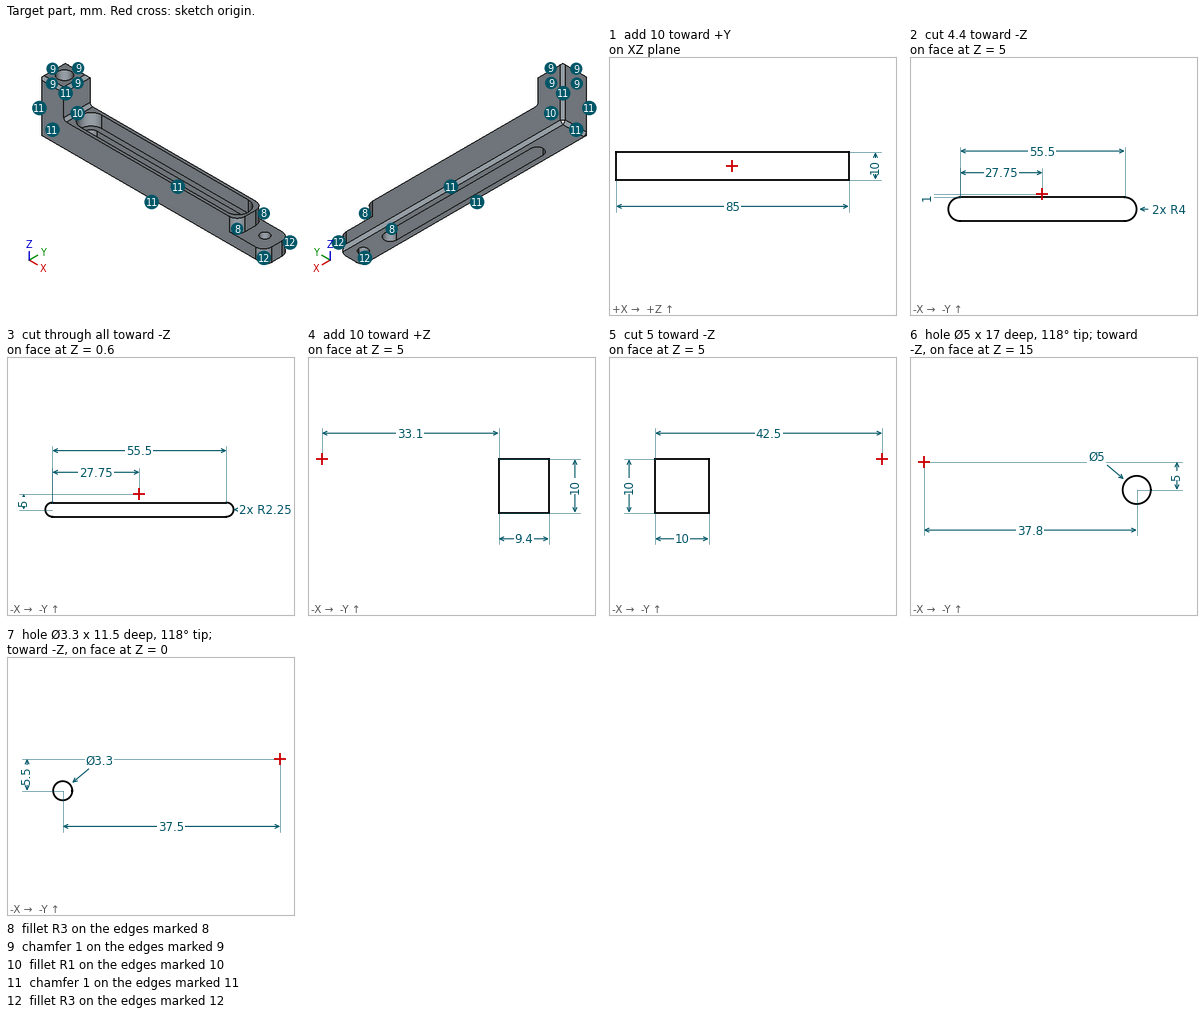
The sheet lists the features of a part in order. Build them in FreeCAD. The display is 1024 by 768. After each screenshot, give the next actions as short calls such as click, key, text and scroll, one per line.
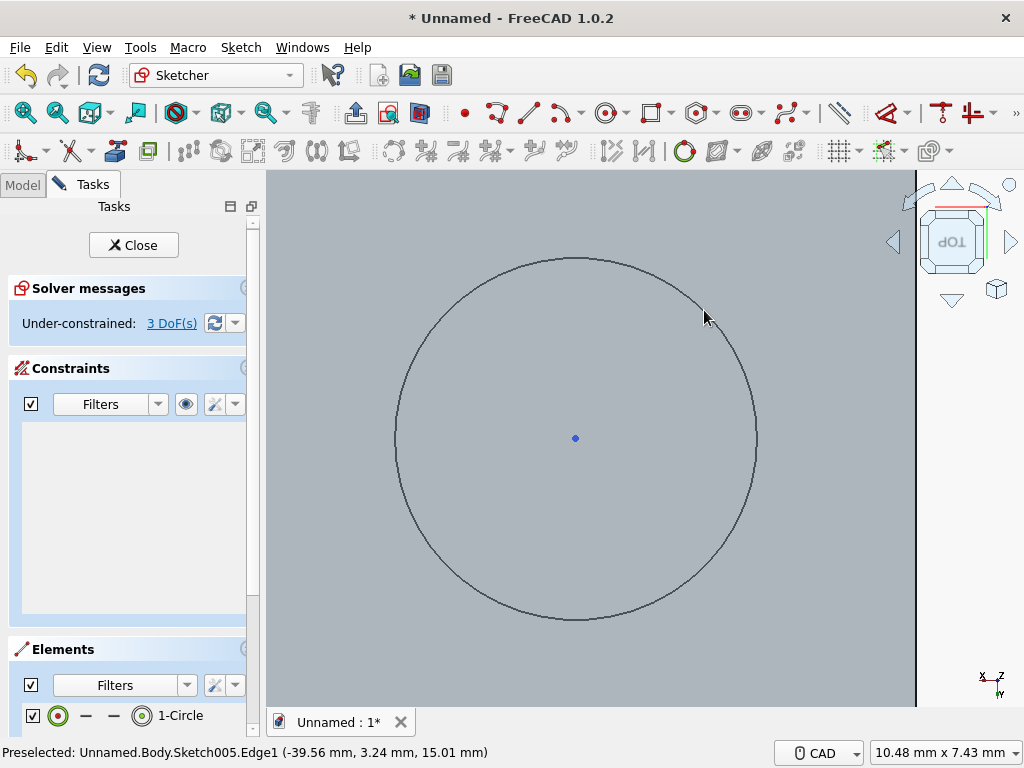
key(d)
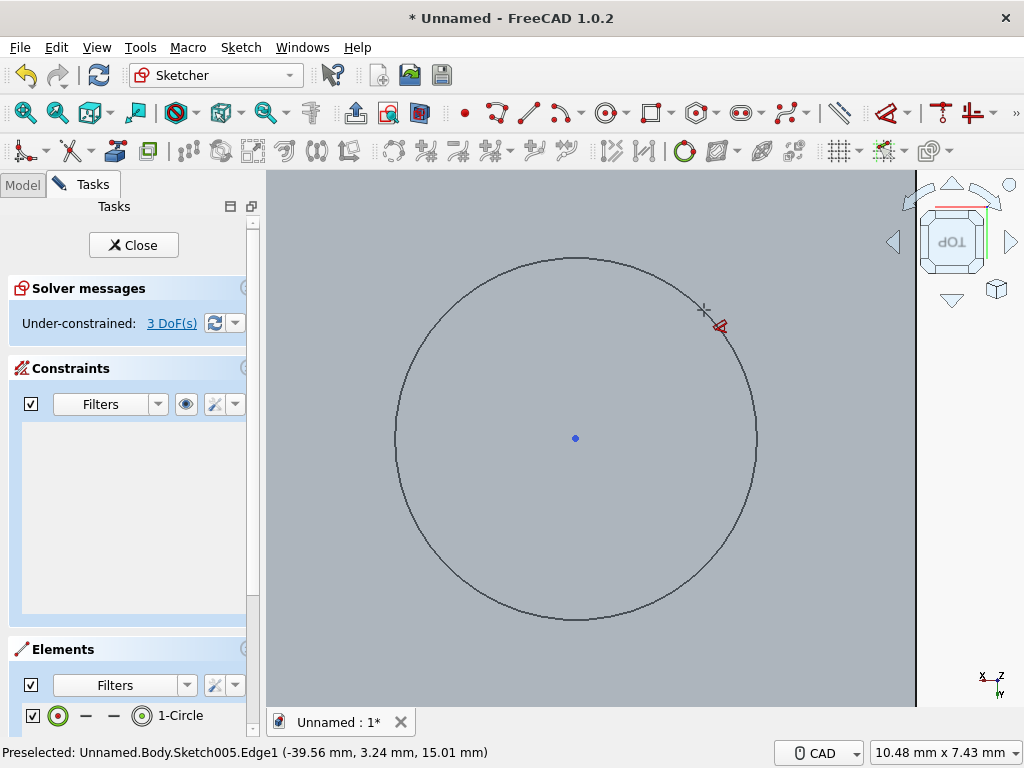
click(704, 311)
click(727, 288)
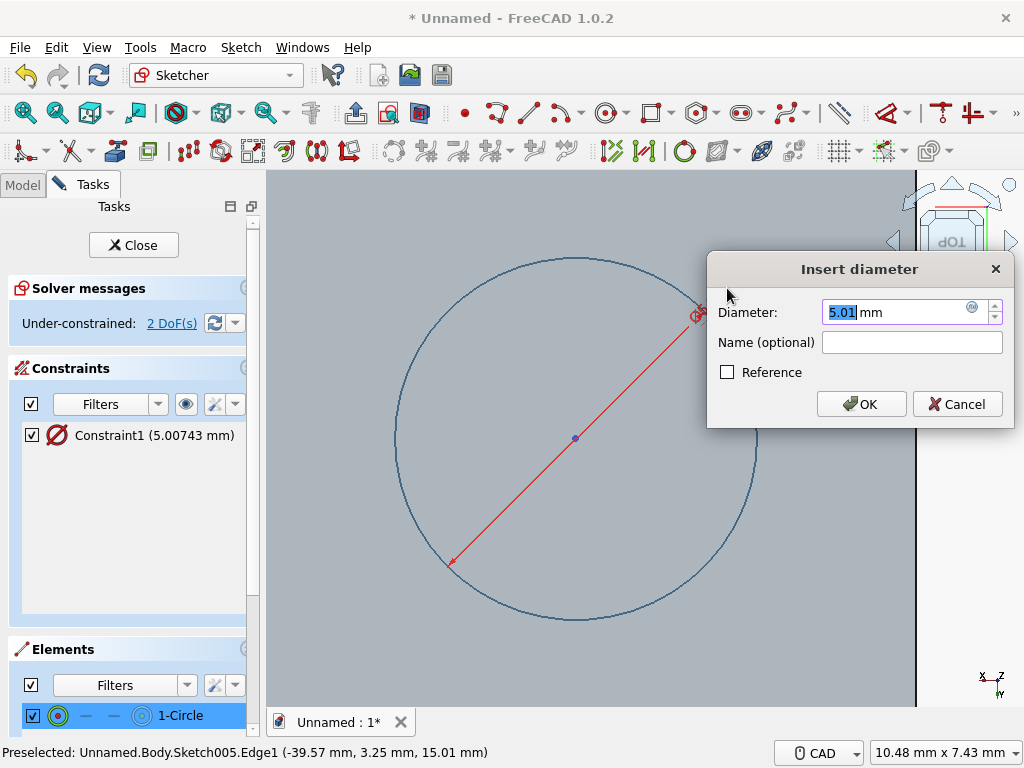
text(5)
key(Return)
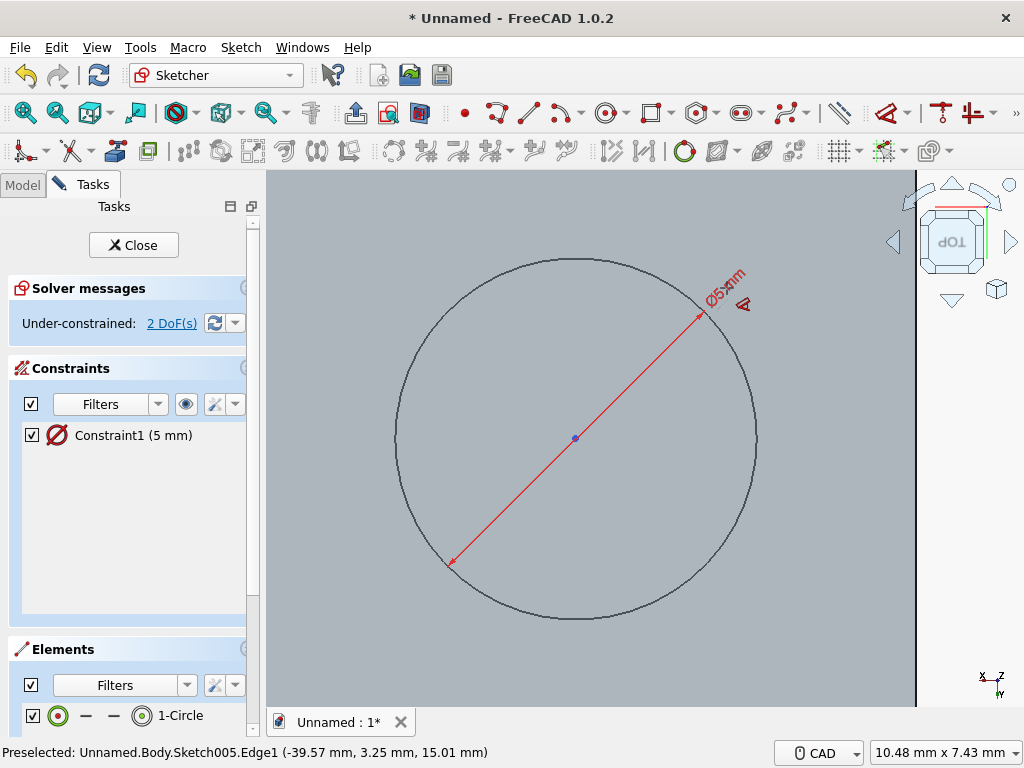
click(576, 439)
click(610, 318)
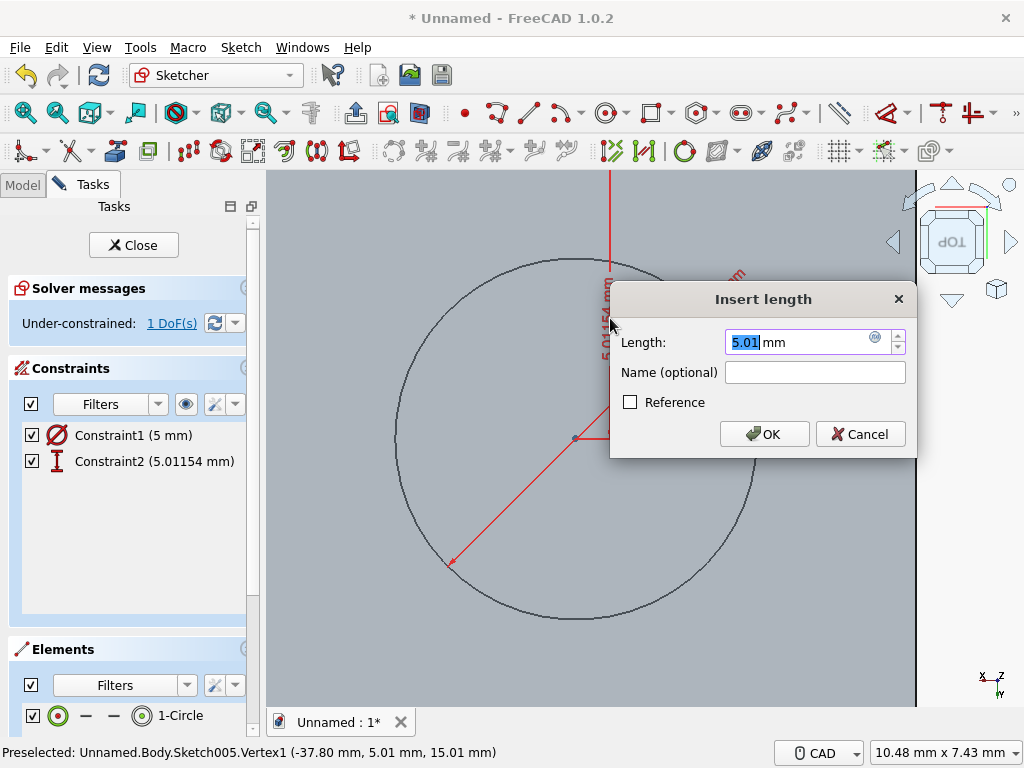
text(5)
key(Return)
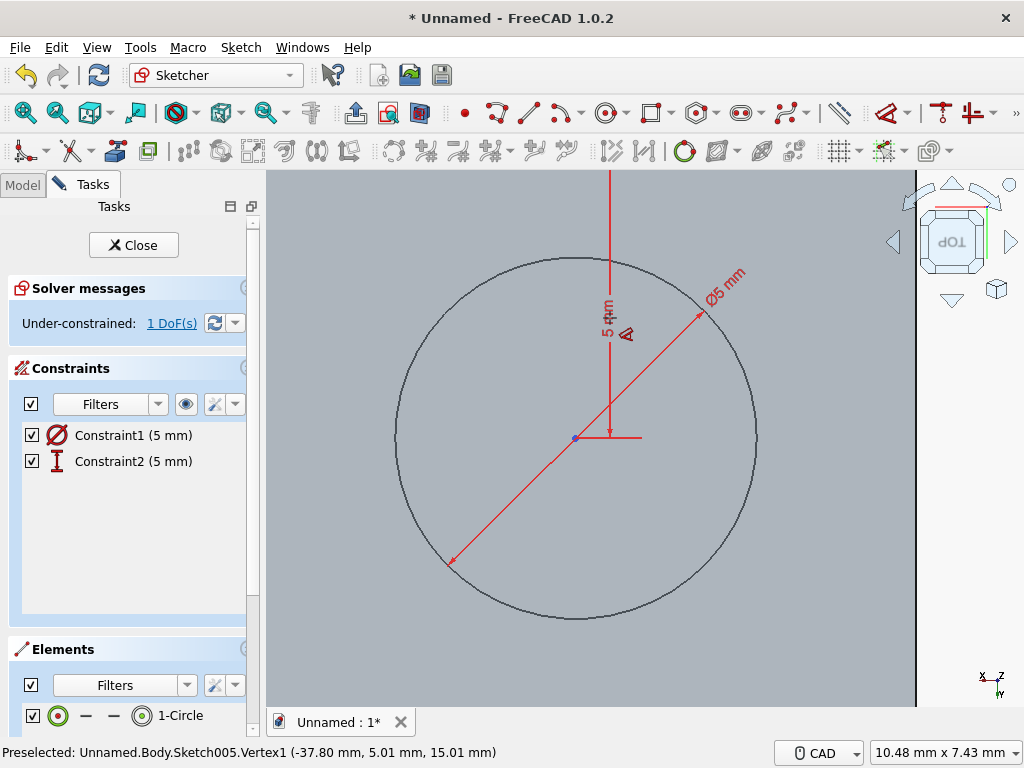
click(576, 438)
click(435, 472)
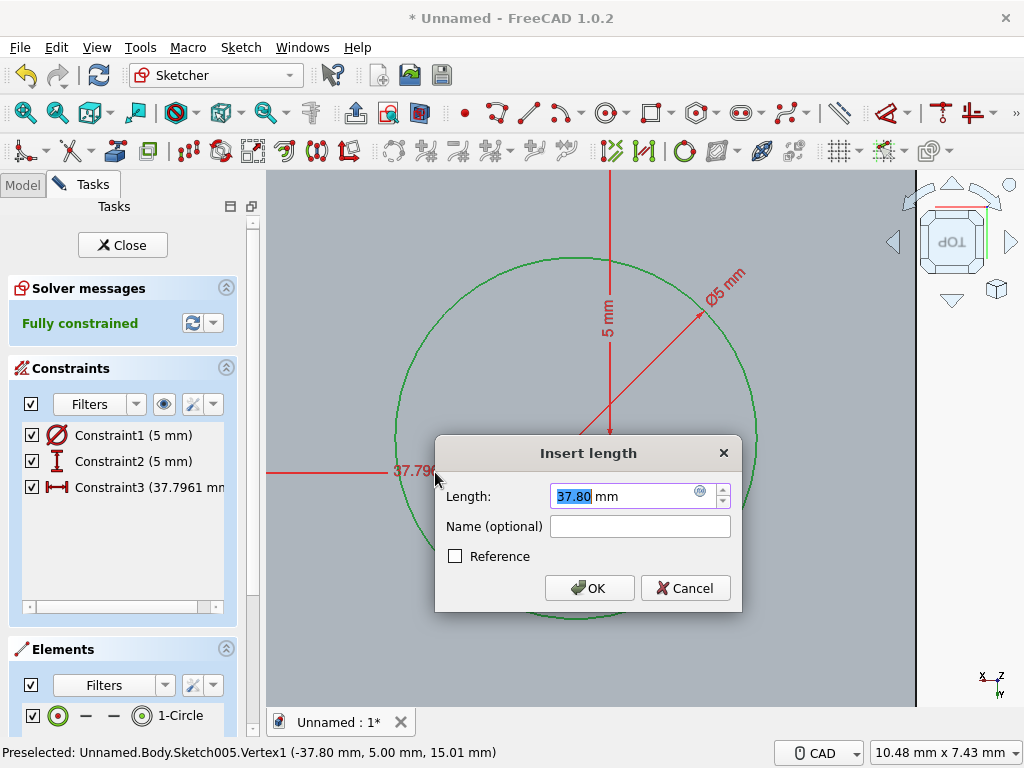
text(37.8)
key(Return)
key(Escape)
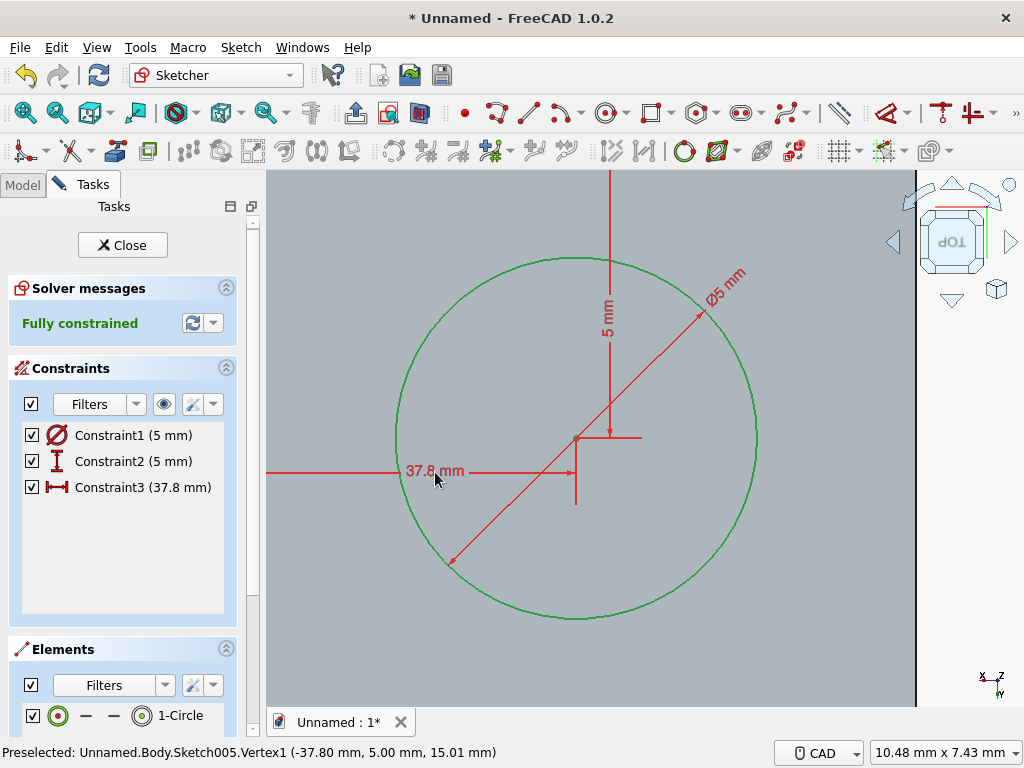
click(123, 245)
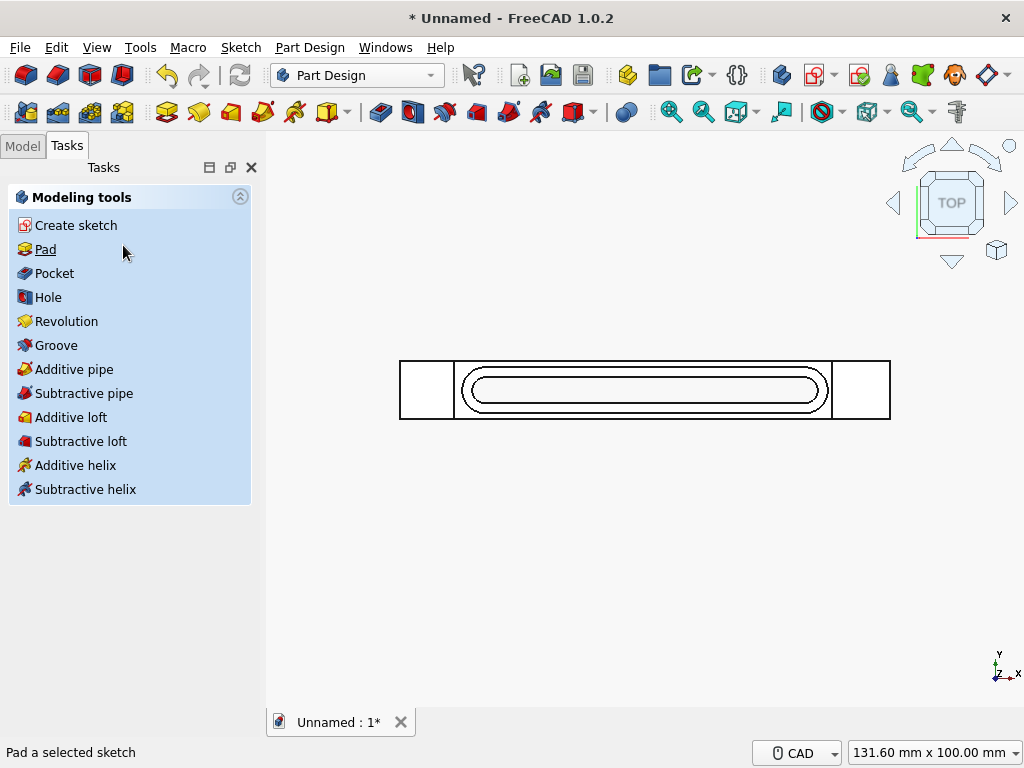
click(414, 112)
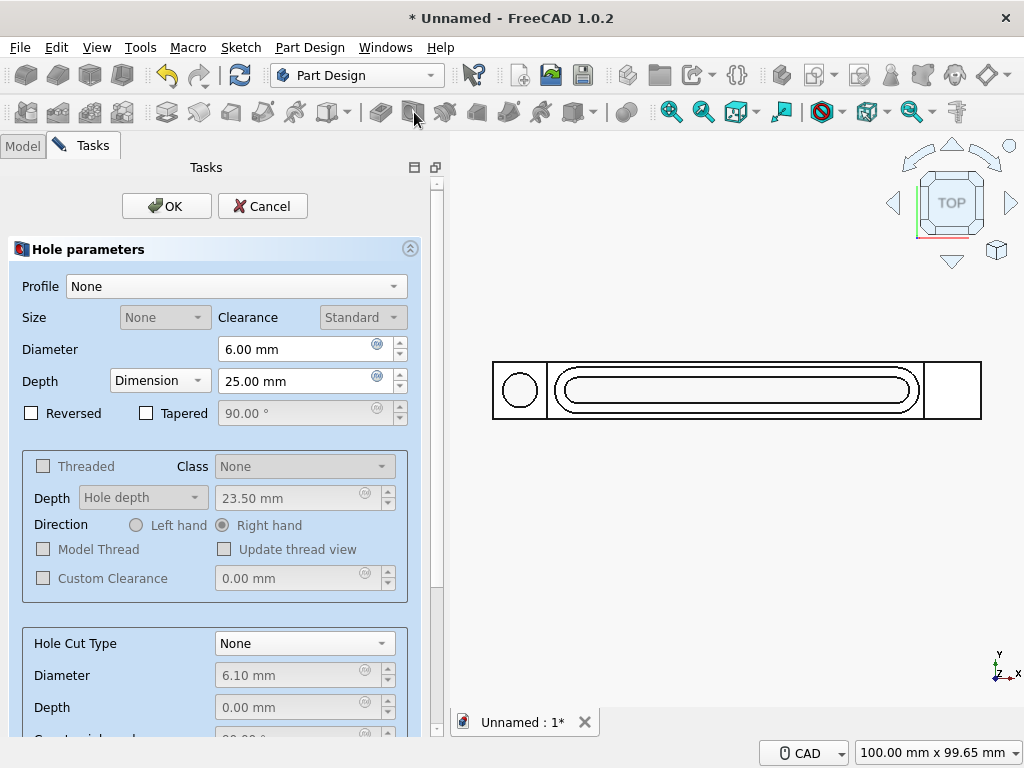
triple_click(305, 349)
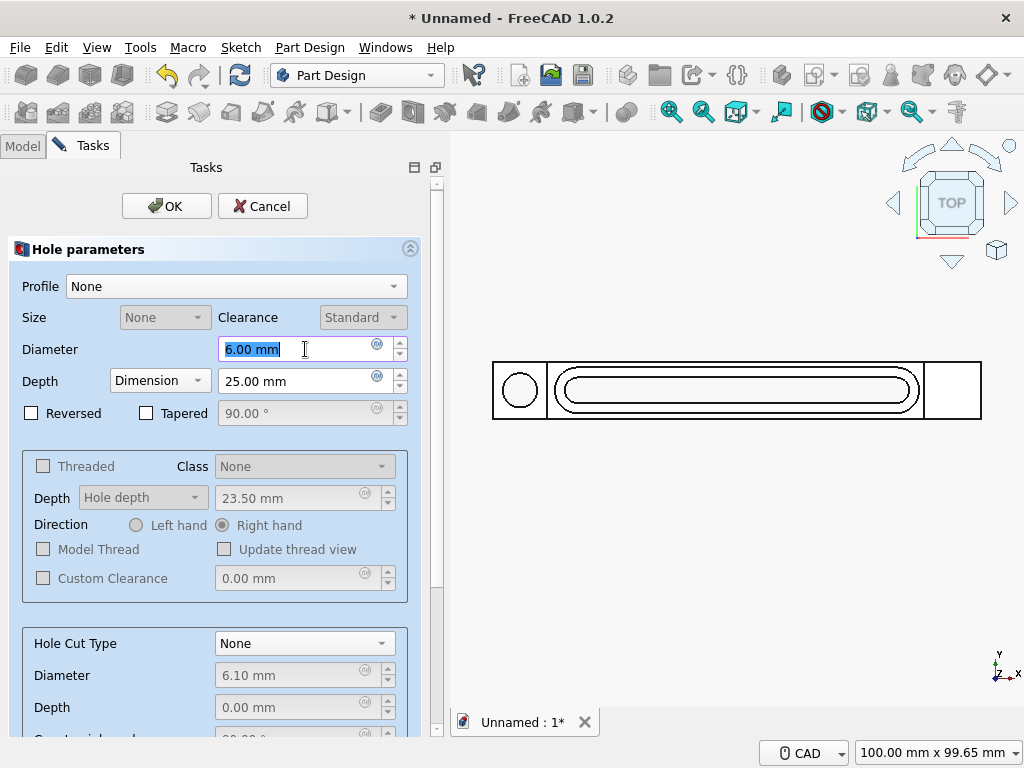
text(5)
key(Tab)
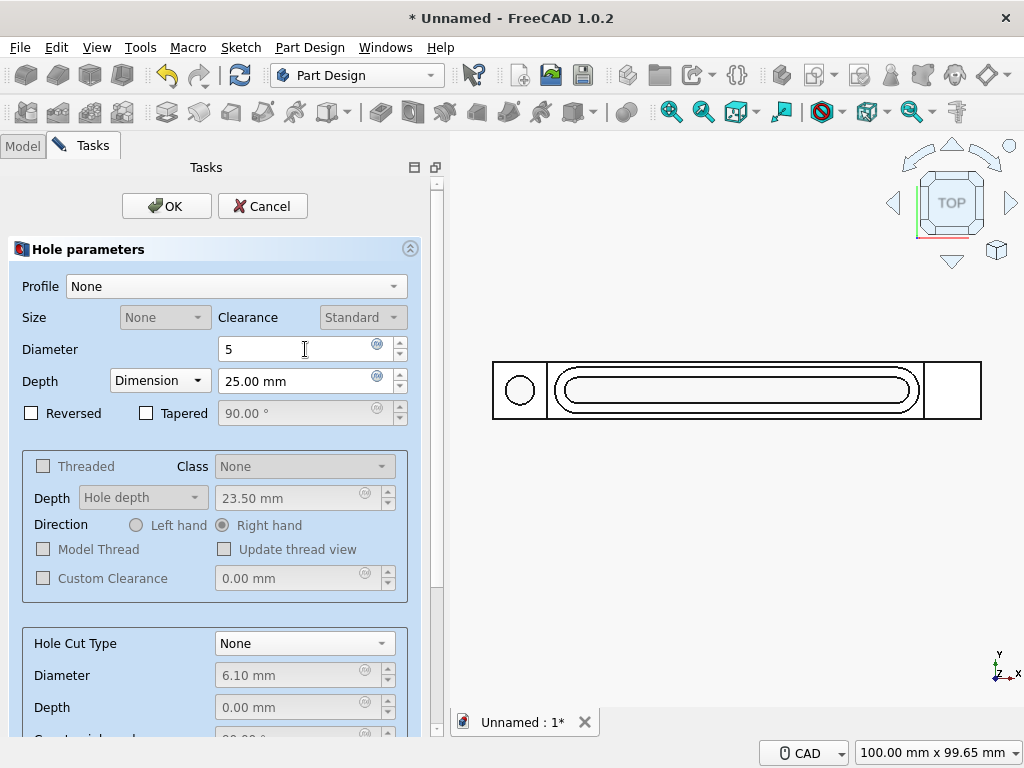
triple_click(305, 381)